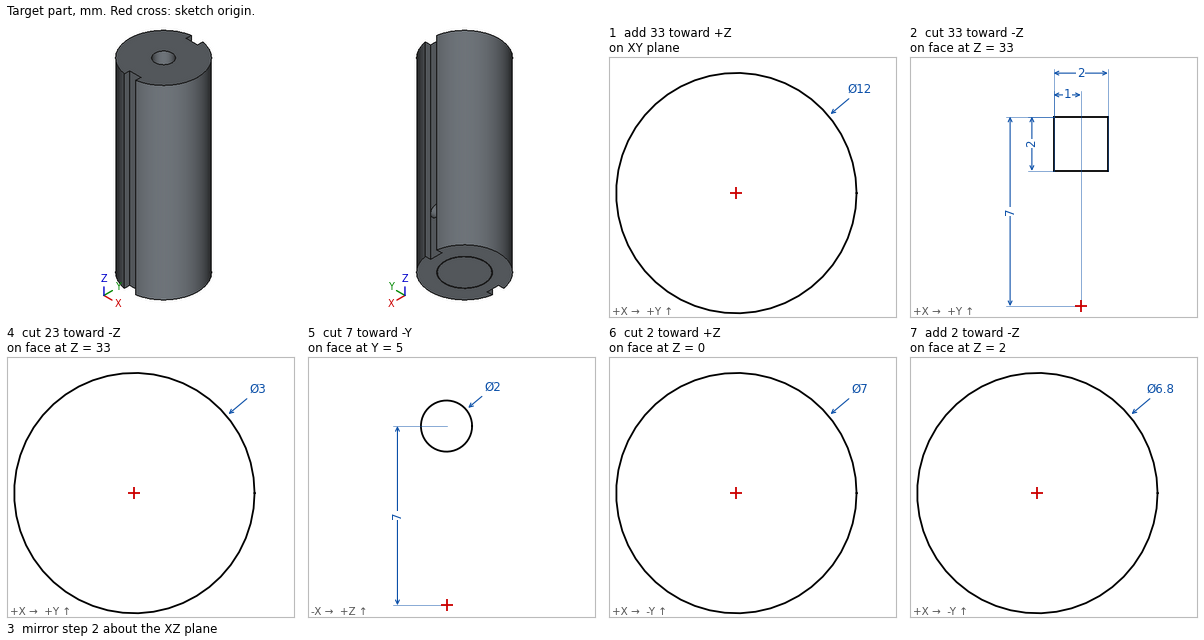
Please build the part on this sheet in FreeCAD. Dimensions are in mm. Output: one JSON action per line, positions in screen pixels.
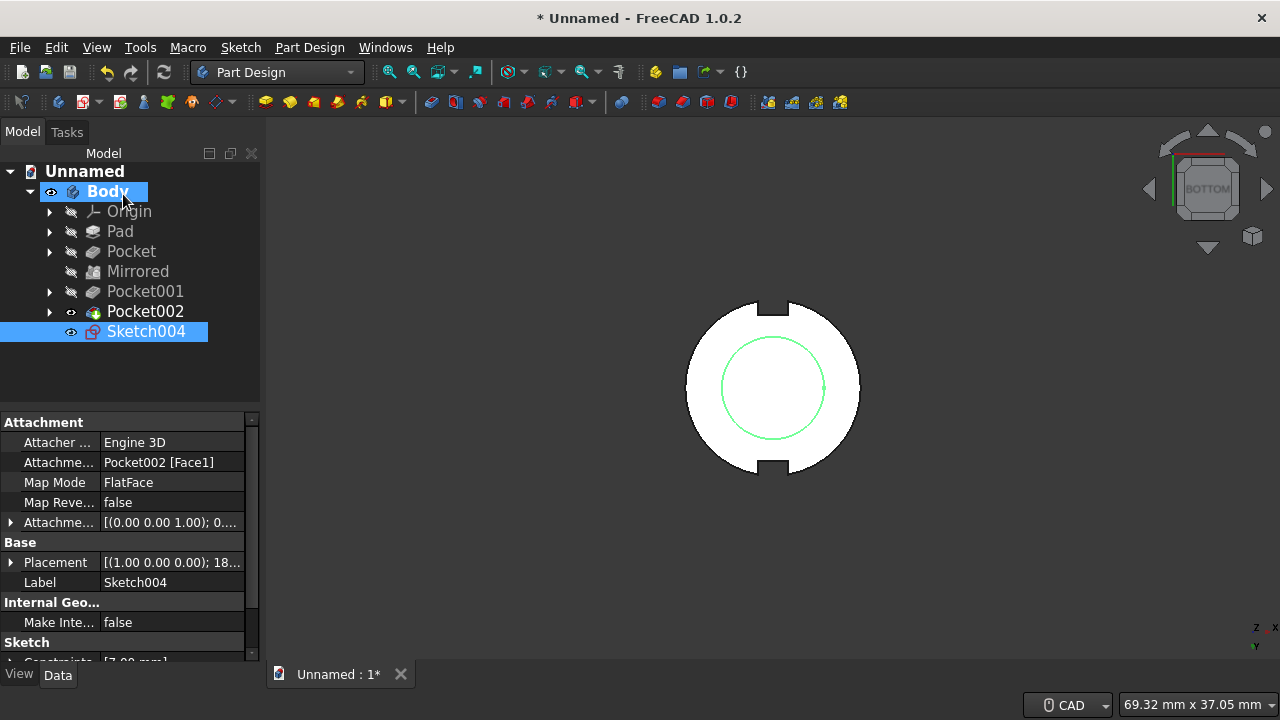
{"action": "left_click", "coordinate": [432, 102]}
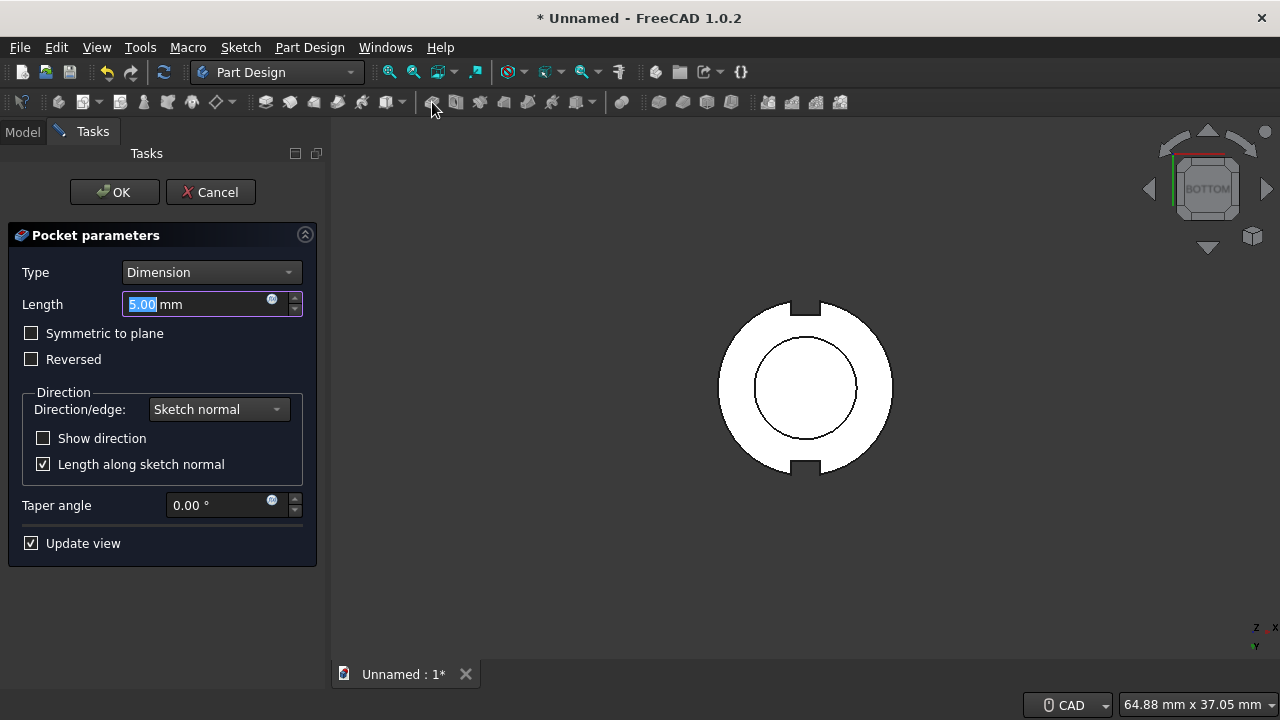
{"action": "type", "text": "2"}
{"action": "key", "text": "Tab"}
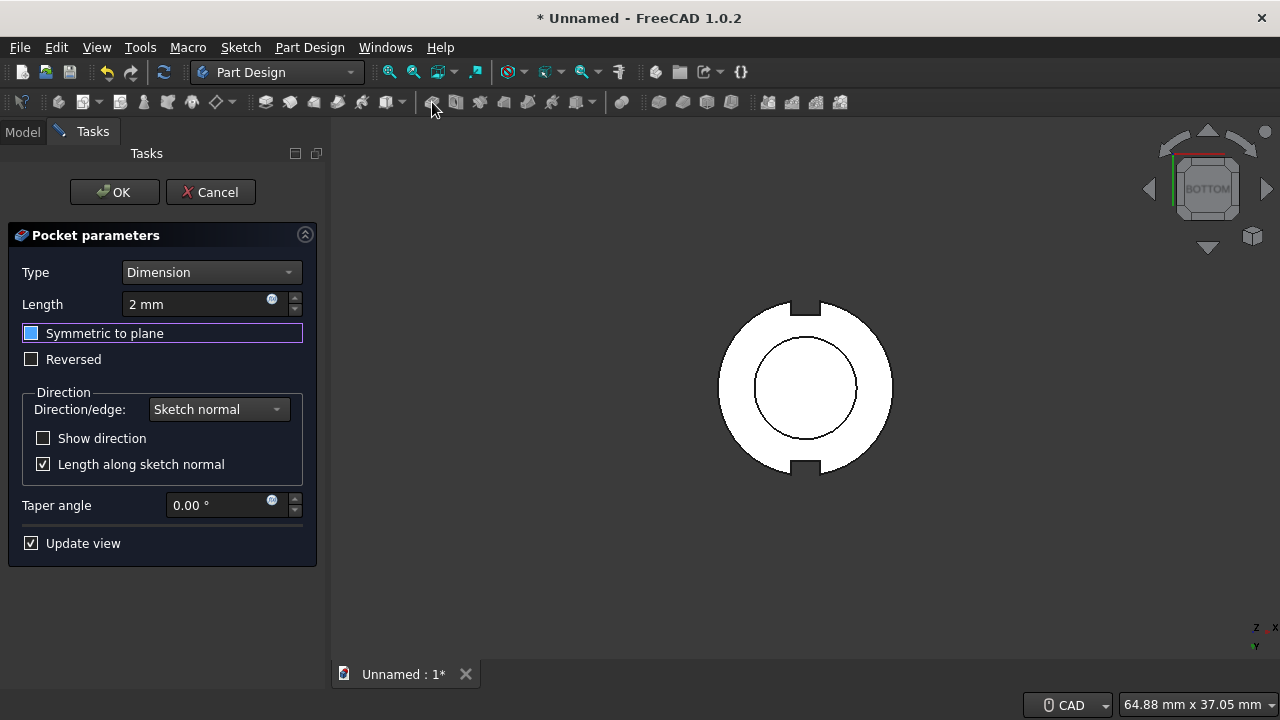
{"action": "left_click", "coordinate": [115, 192]}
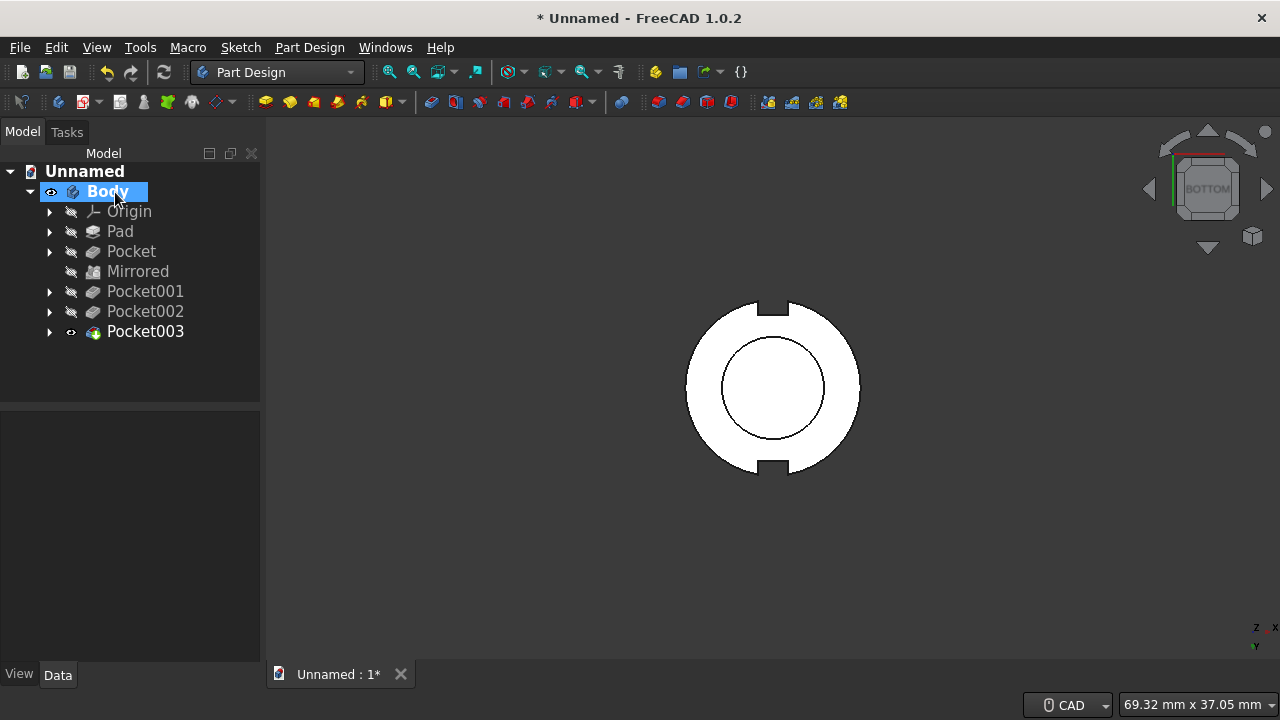
{"action": "left_click", "coordinate": [390, 72]}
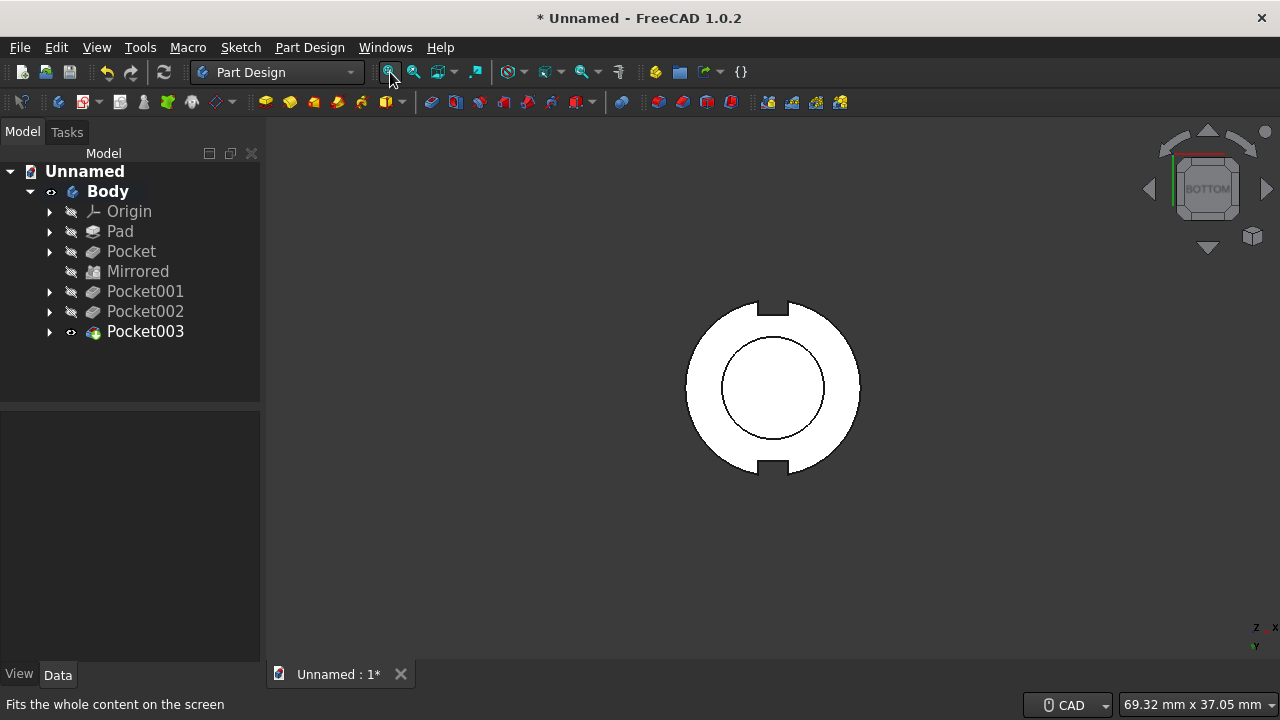
{"action": "left_click", "coordinate": [773, 387]}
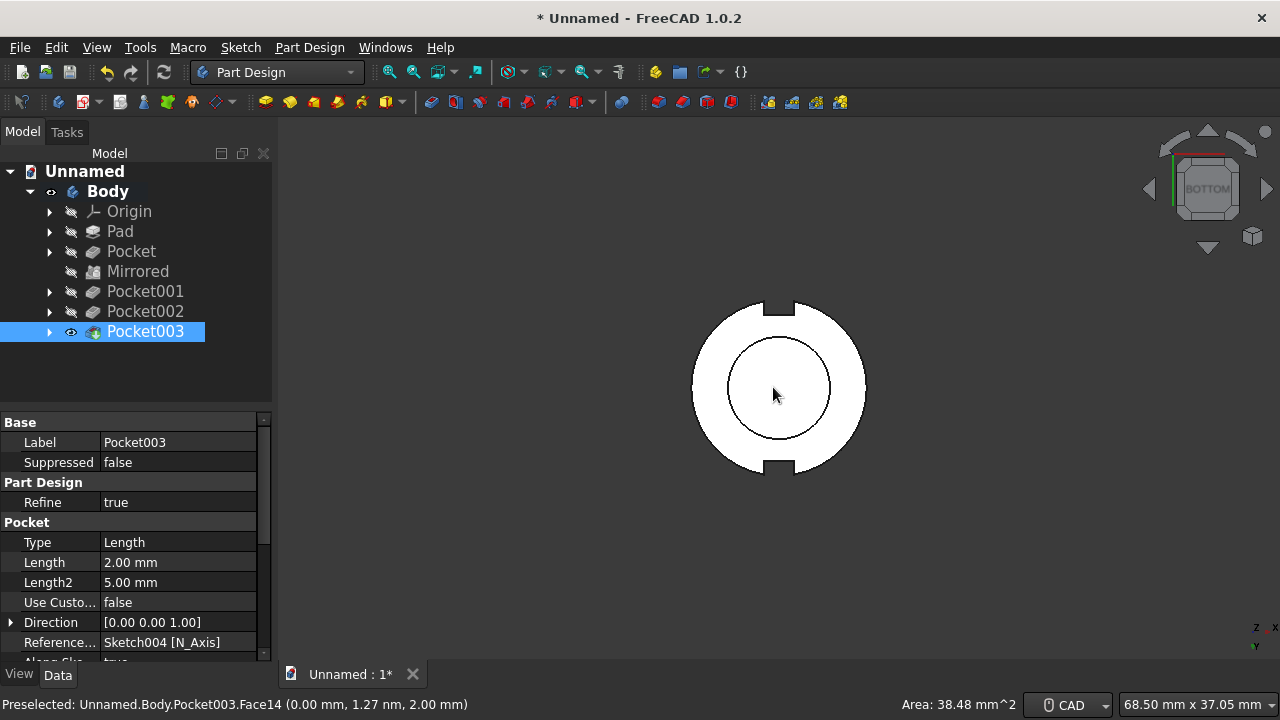
{"action": "left_click", "coordinate": [84, 102]}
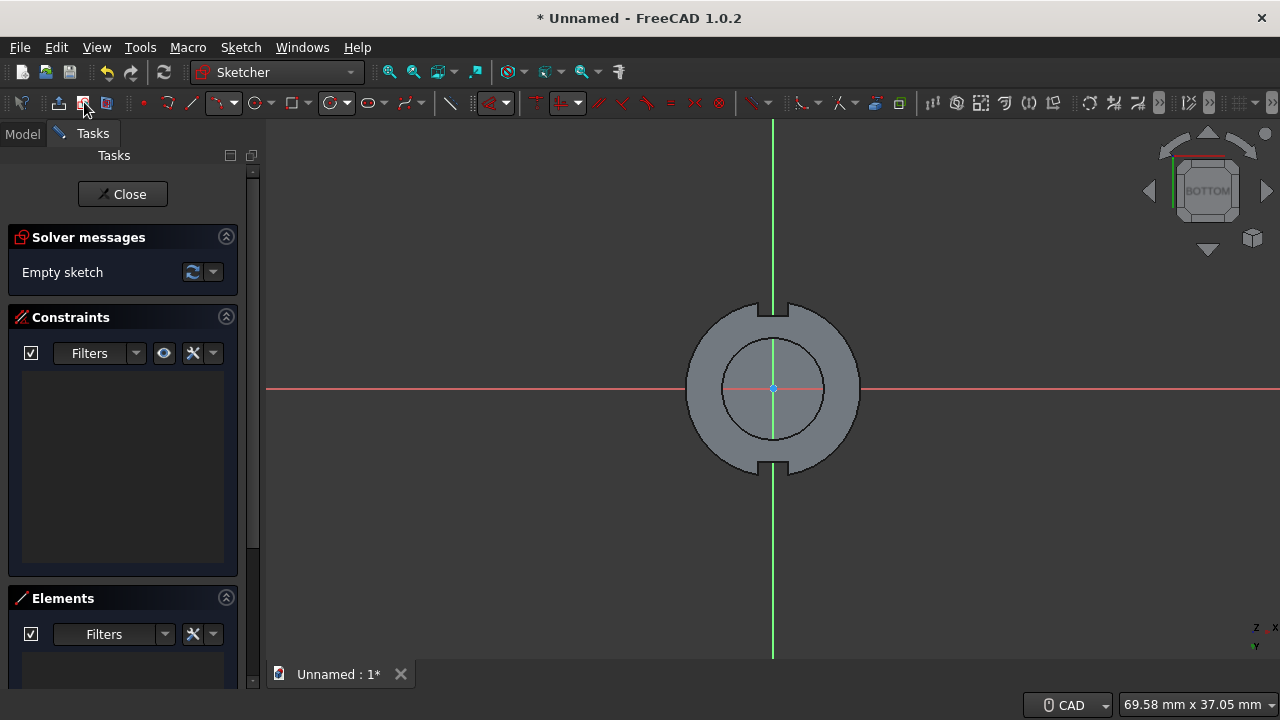
{"action": "key", "text": "q s"}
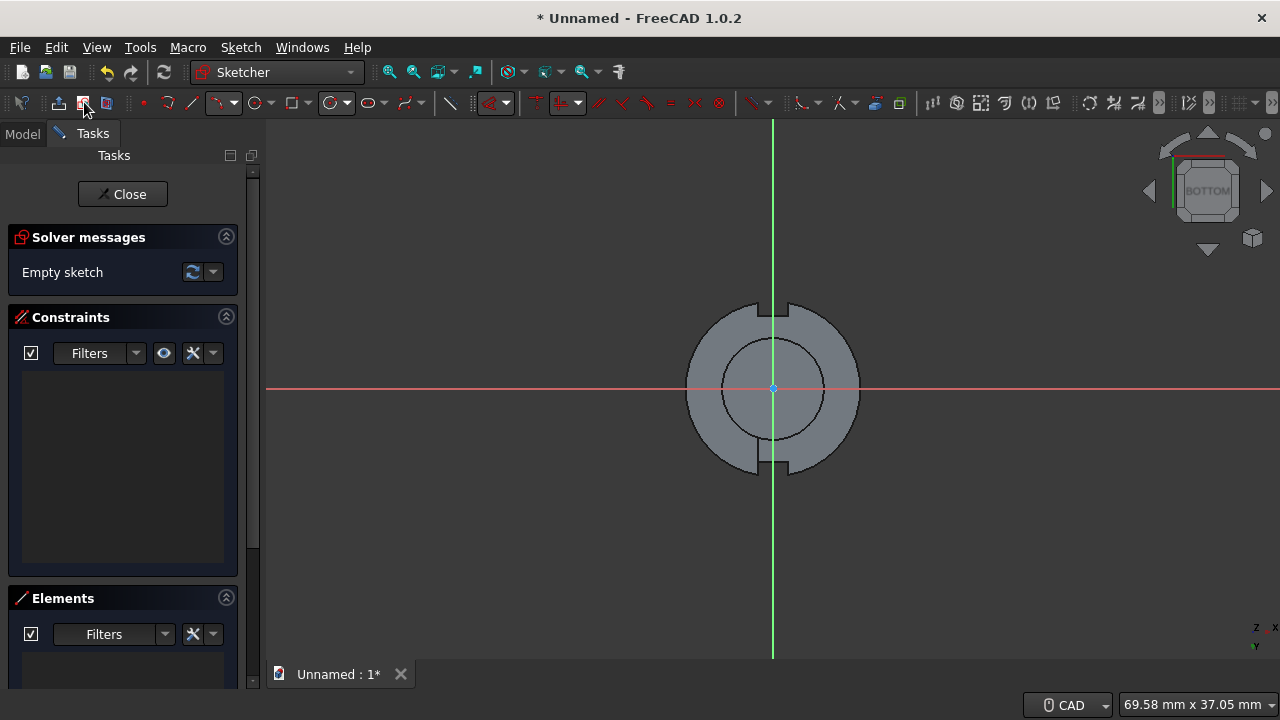
{"action": "scroll", "coordinate": [803, 389], "scroll_direction": "up", "scroll_amount": 6}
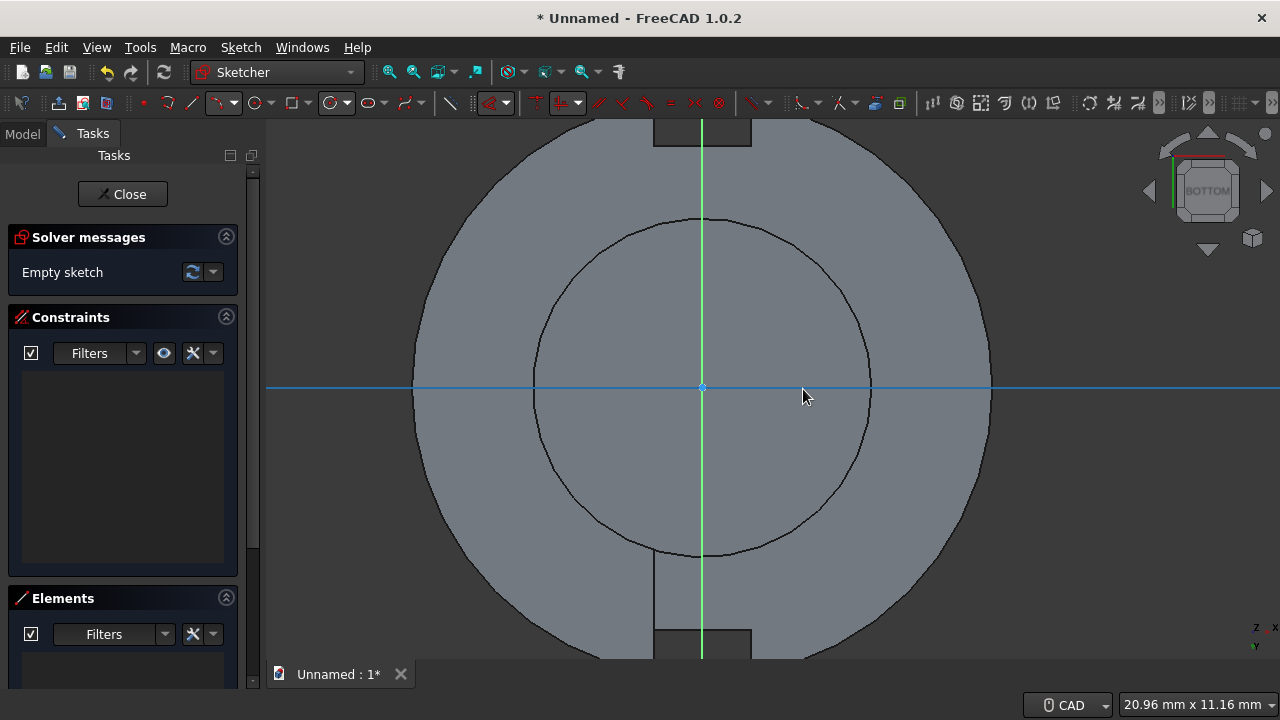
{"action": "key", "text": "g c"}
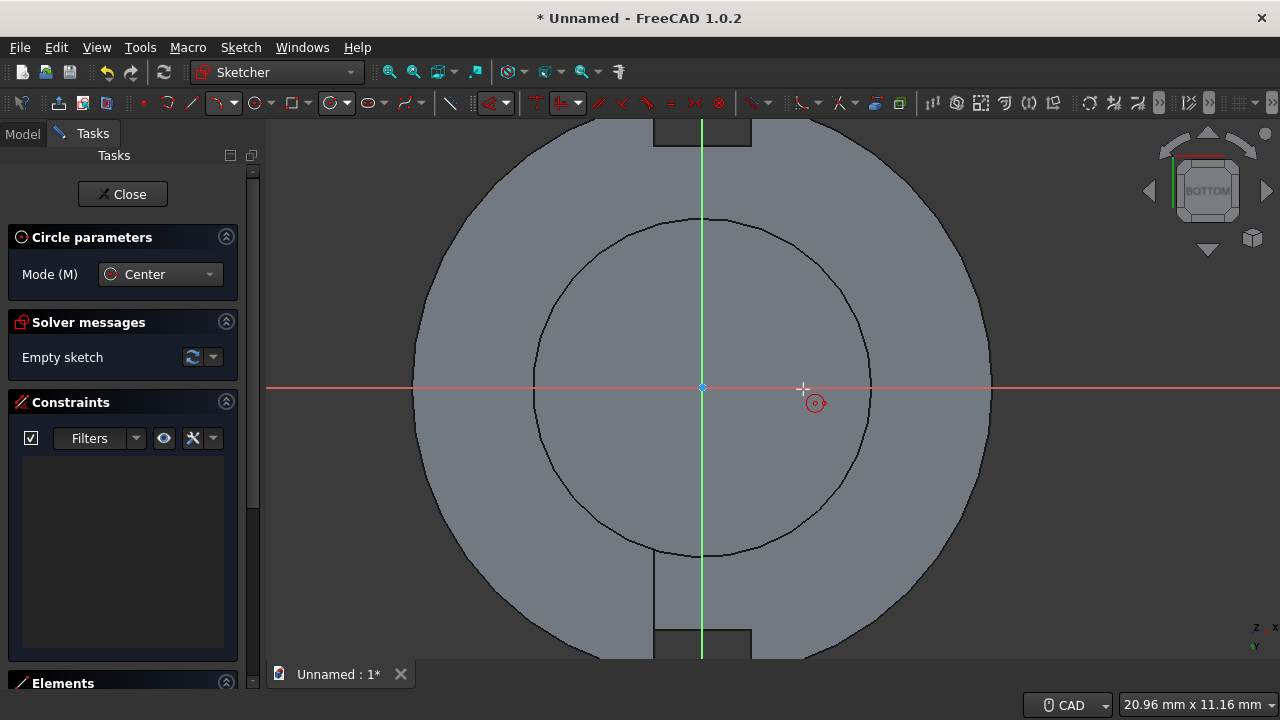
{"action": "left_click", "coordinate": [702, 388]}
{"action": "left_click", "coordinate": [818, 272]}
{"action": "key", "text": "Escape"}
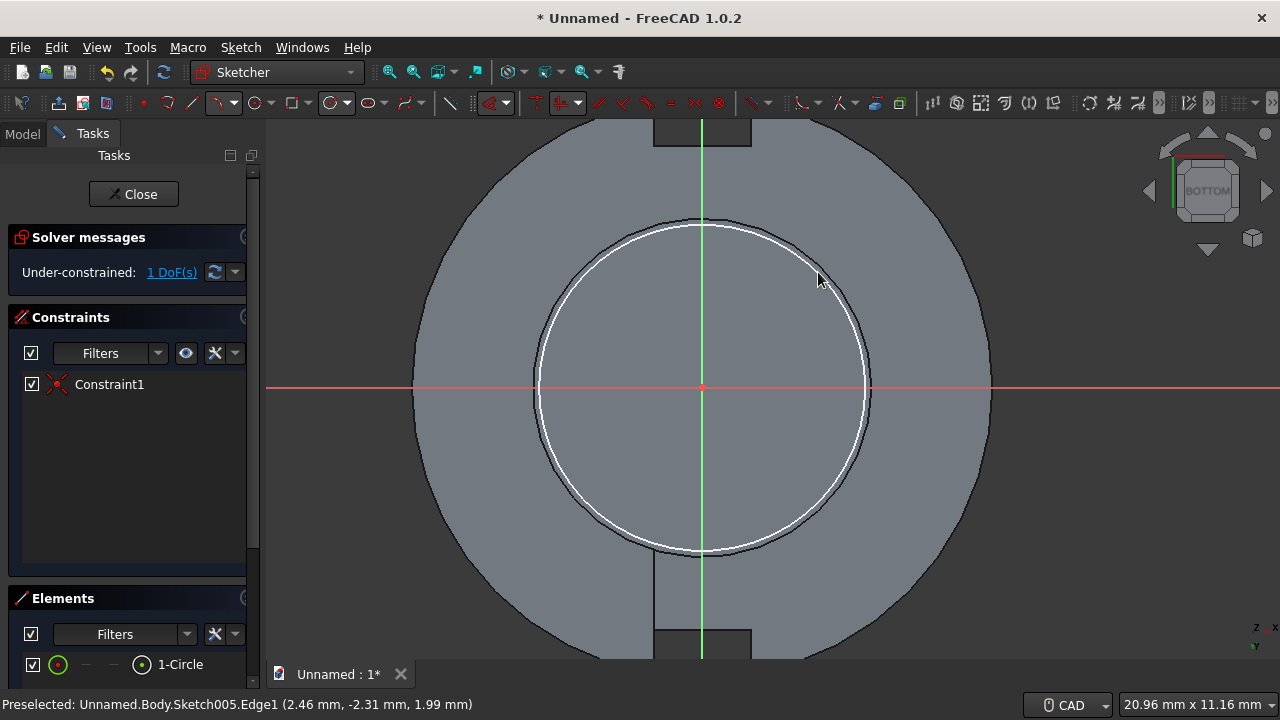
{"action": "left_click", "coordinate": [490, 104]}